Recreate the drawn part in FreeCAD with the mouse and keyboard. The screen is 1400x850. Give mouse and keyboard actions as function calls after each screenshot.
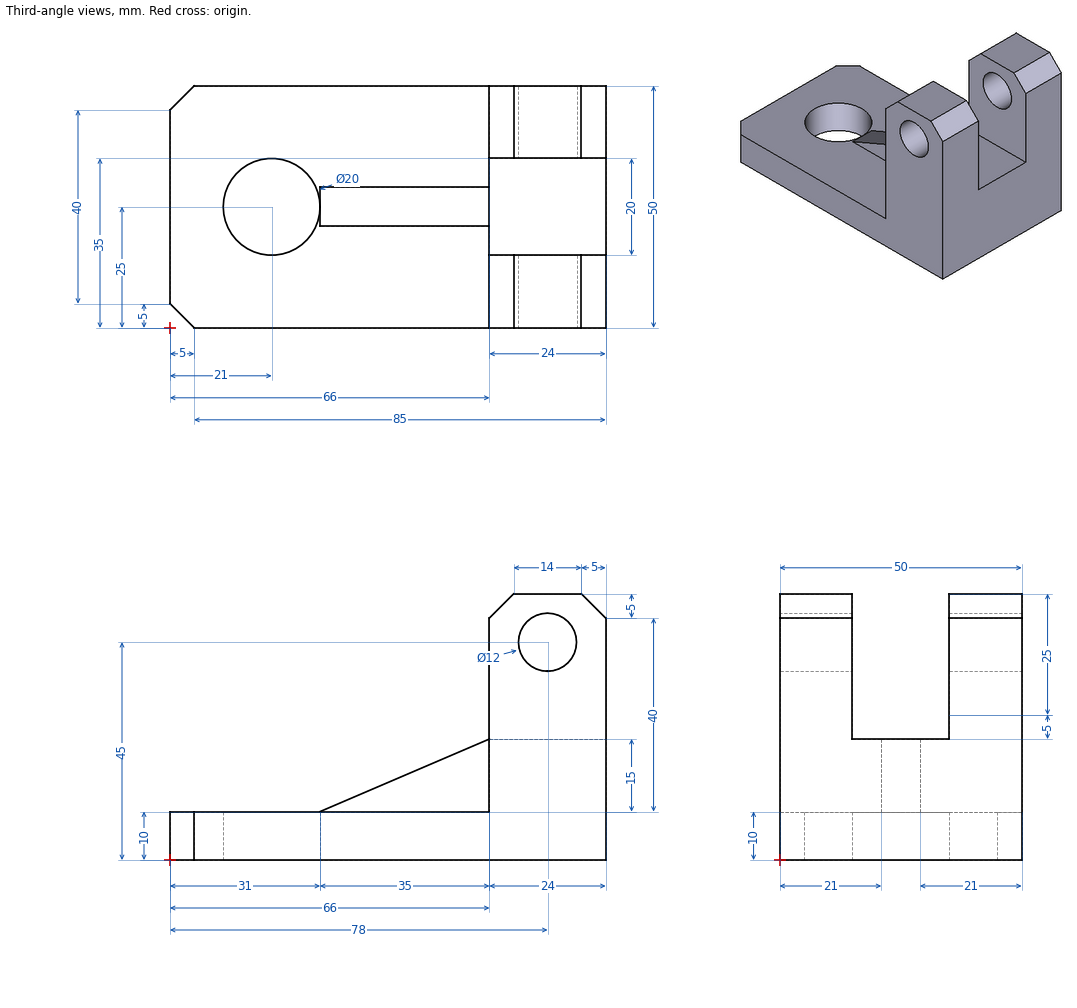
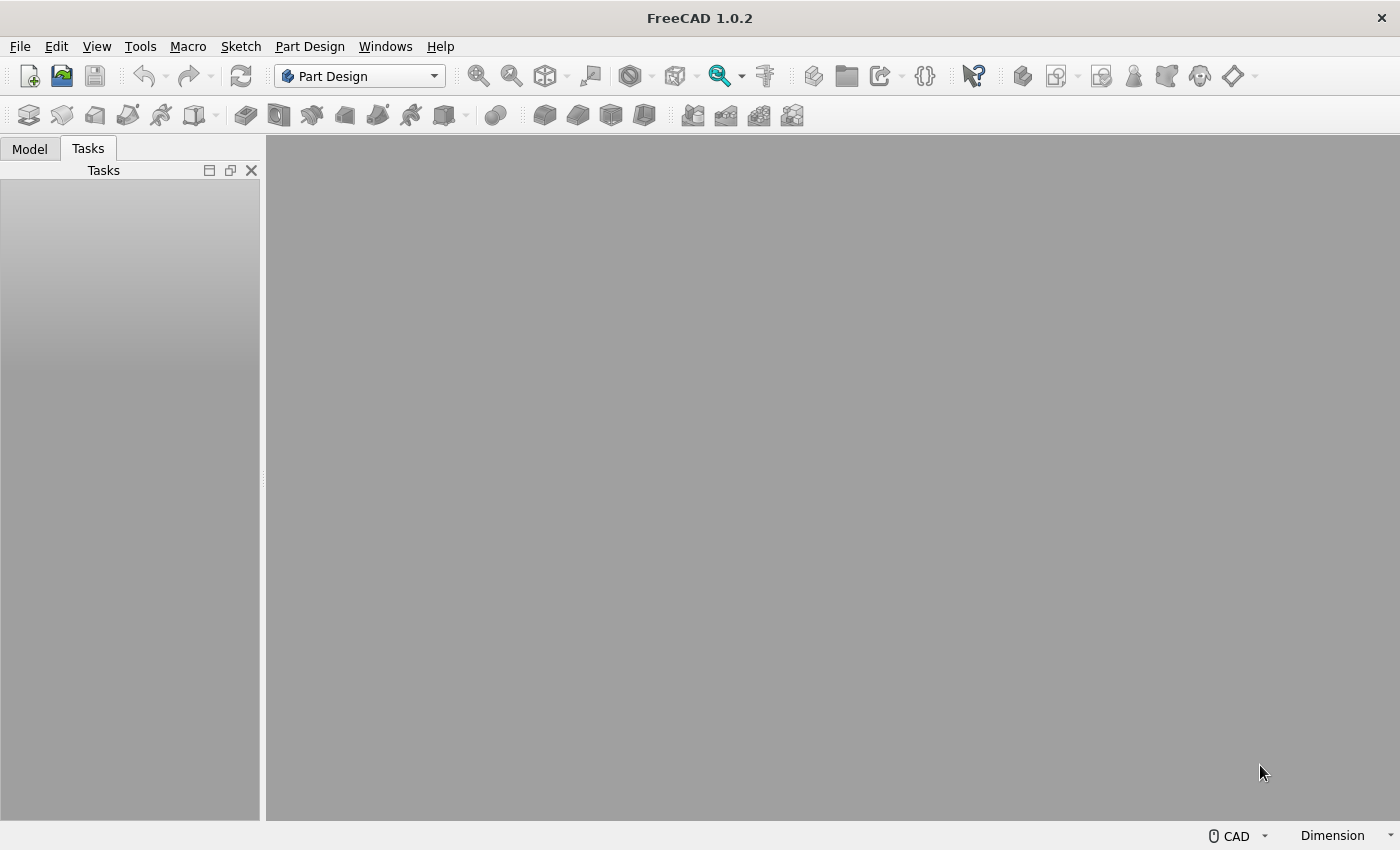
click(29, 76)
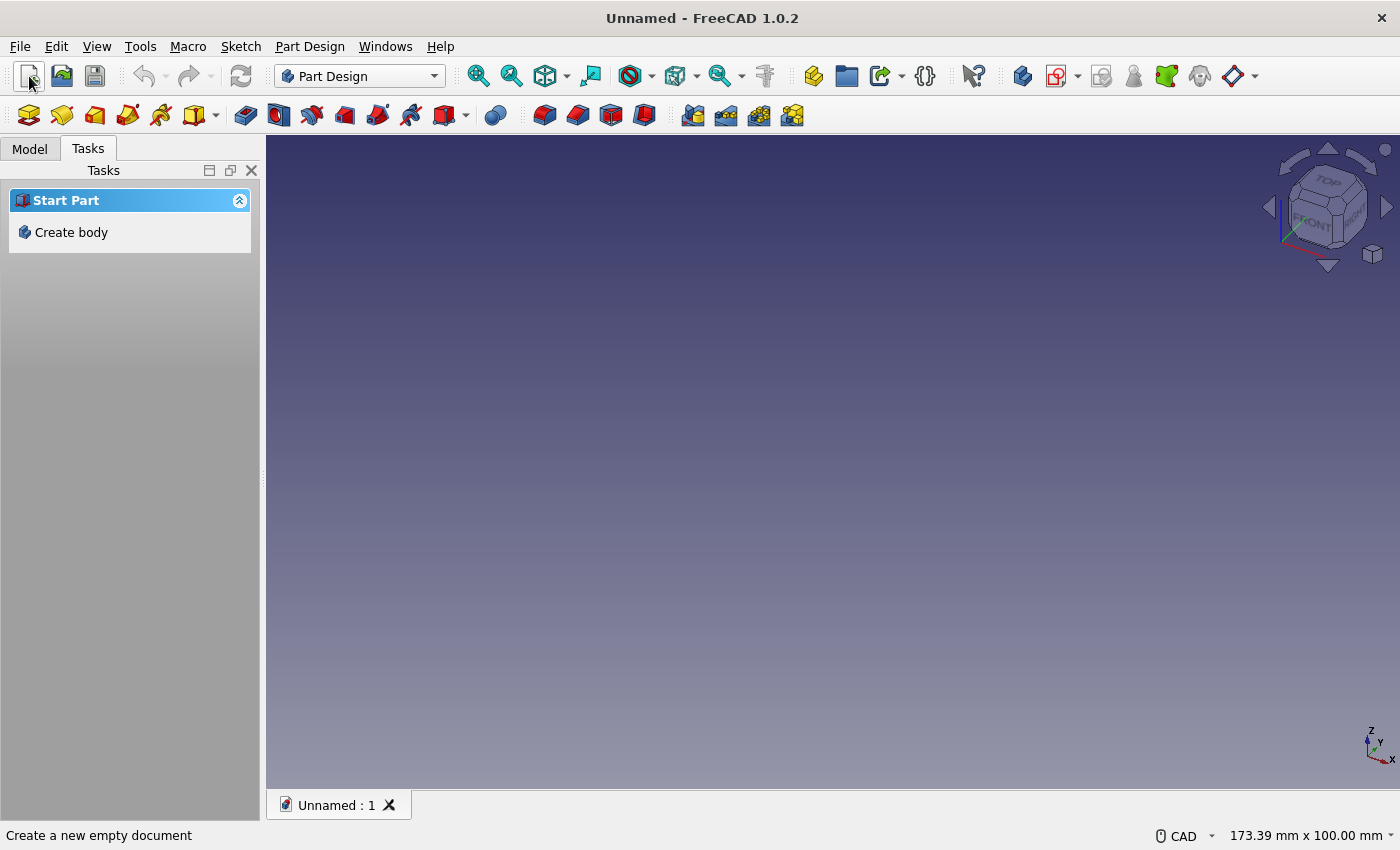
click(1056, 76)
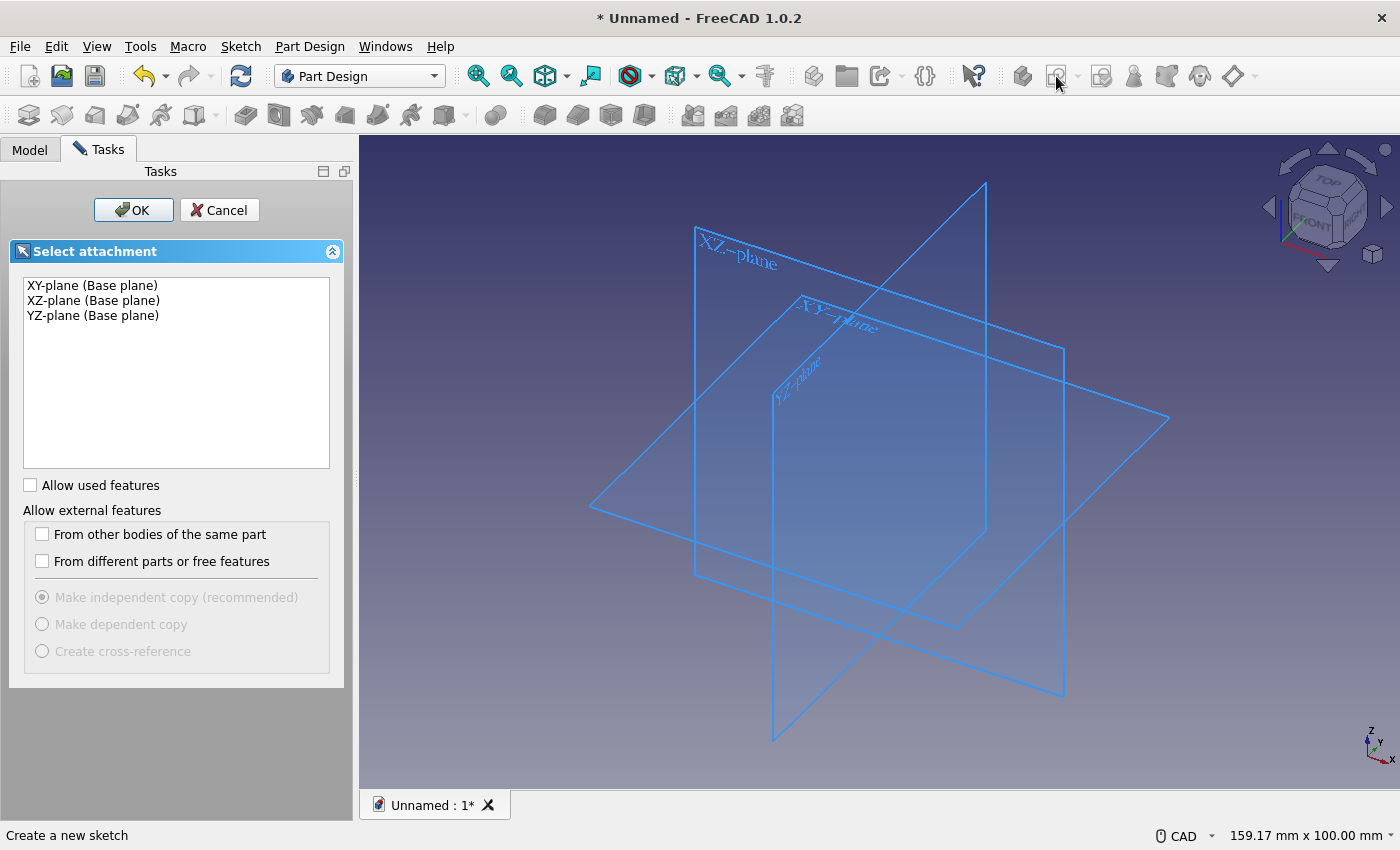
click(84, 286)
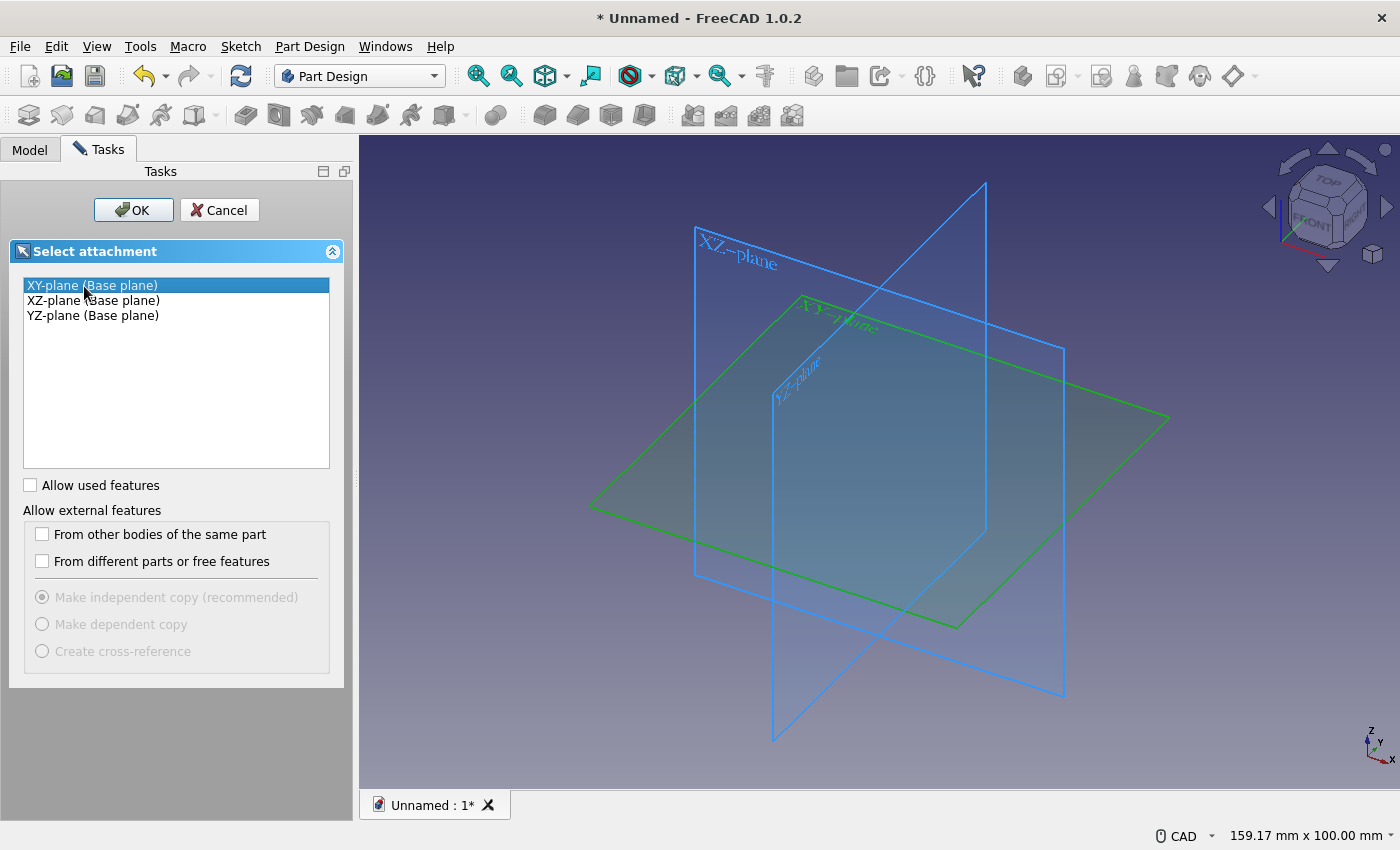
click(134, 210)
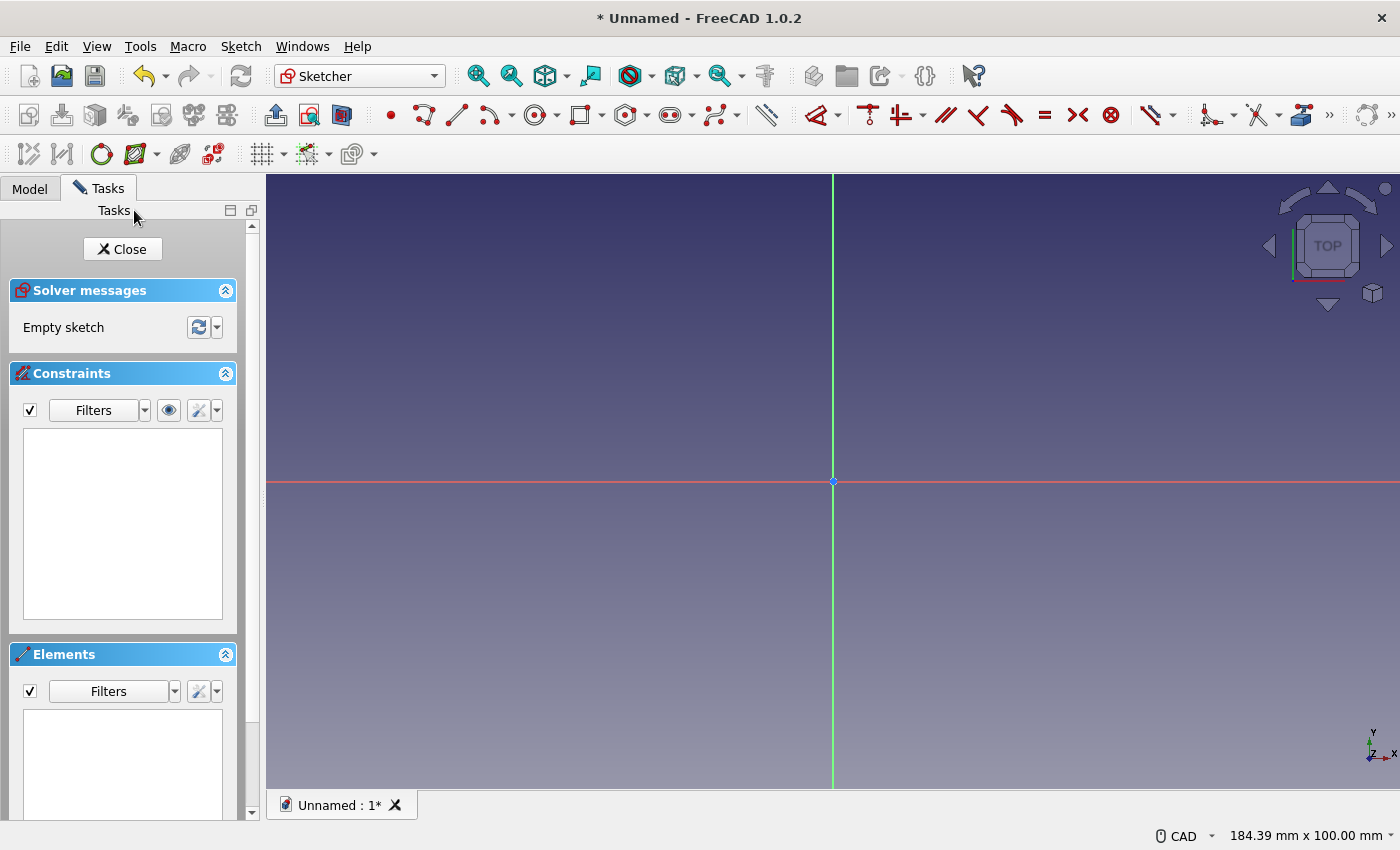
scroll(294, 761, down, 1)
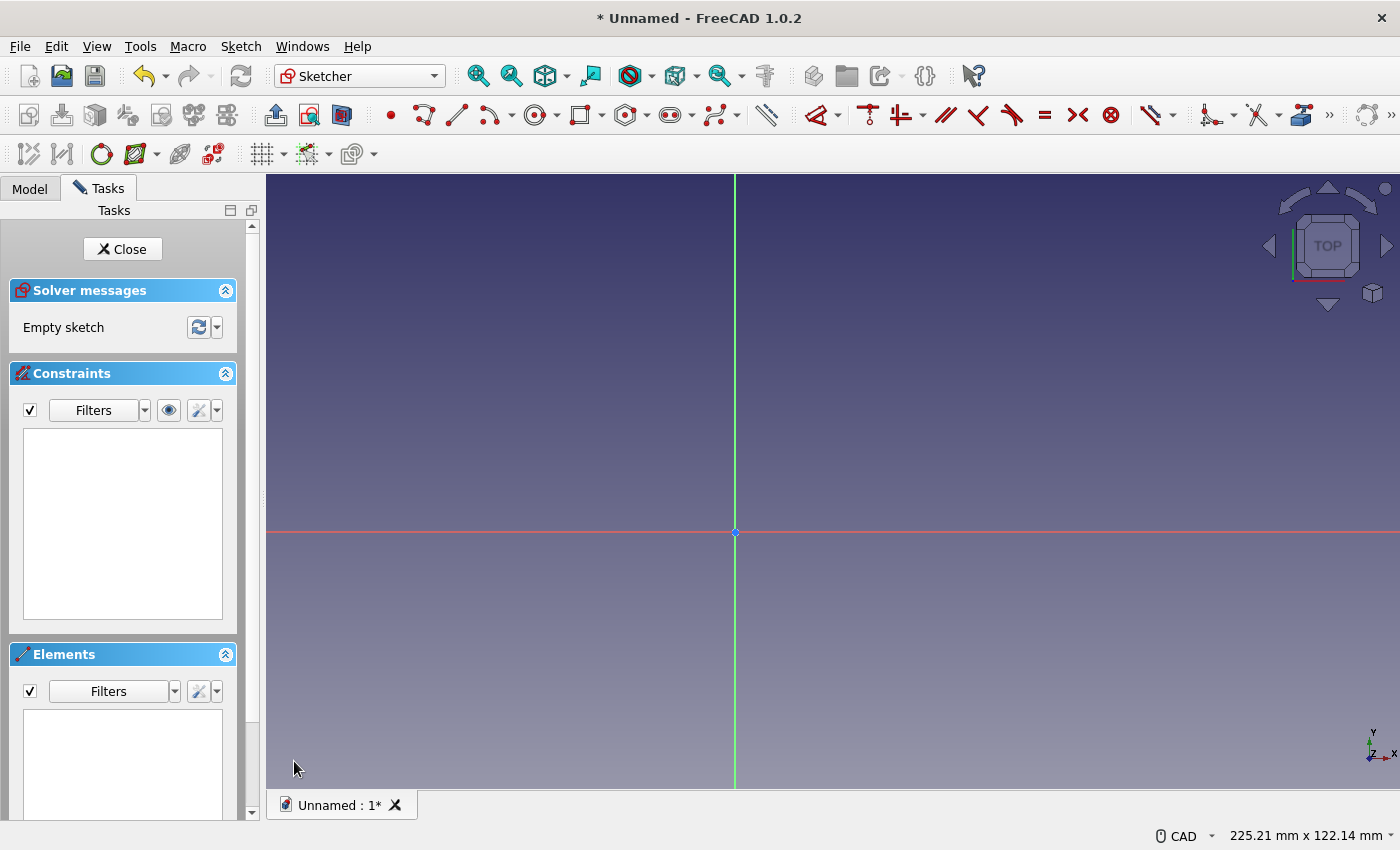
scroll(1235, 254, up, 2)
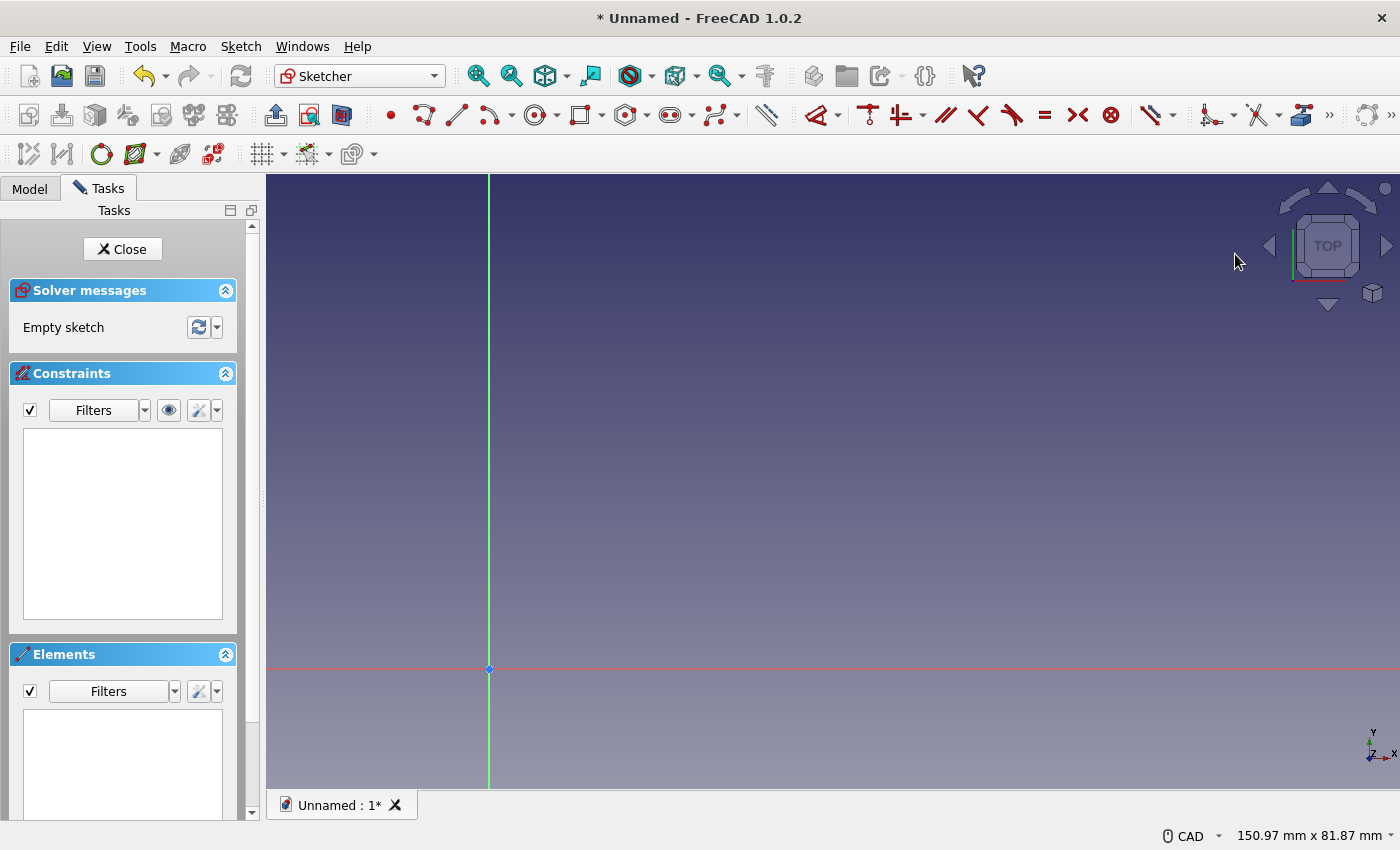
click(424, 116)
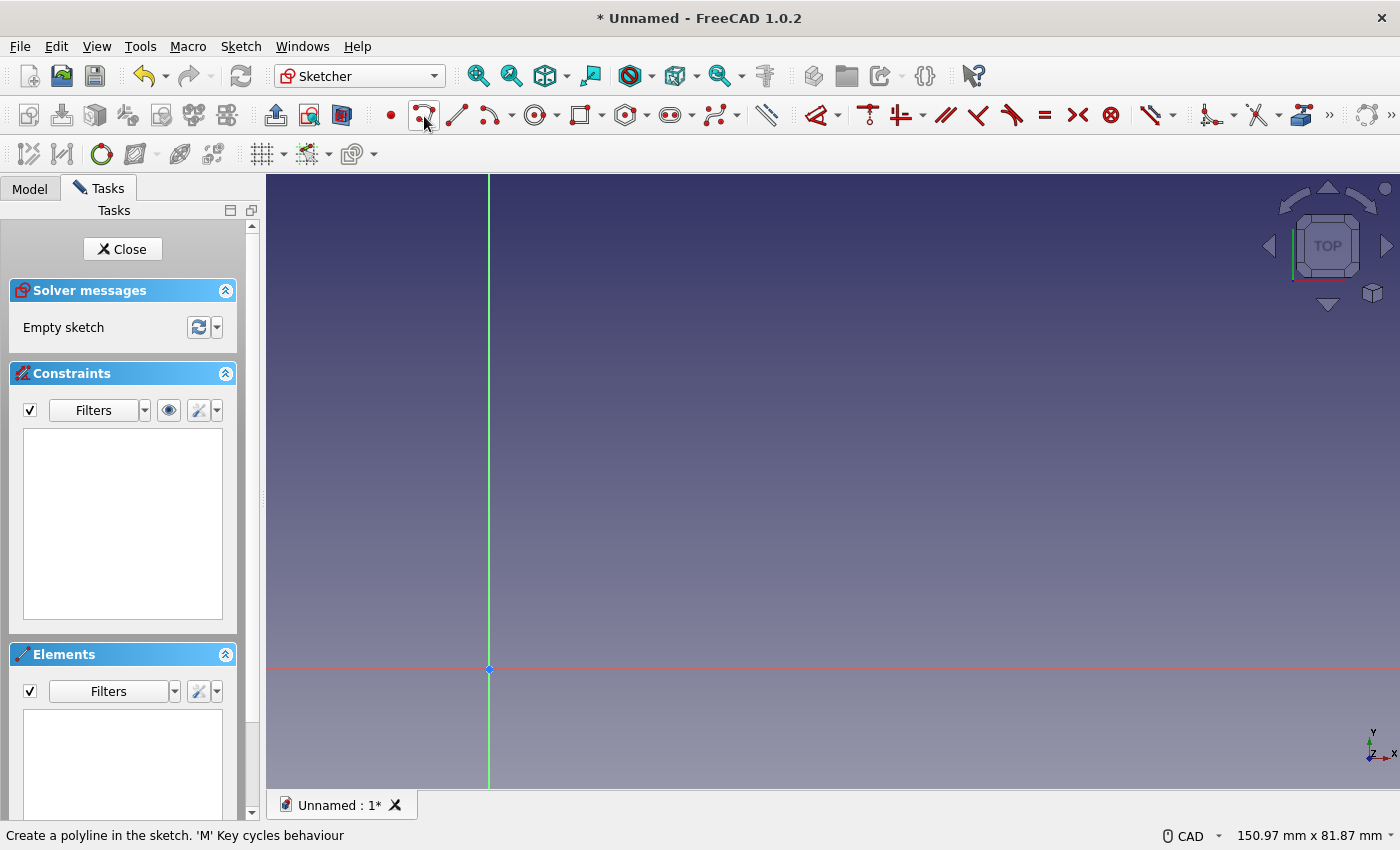
click(527, 669)
click(1165, 660)
click(1165, 294)
click(527, 294)
click(489, 331)
click(498, 632)
click(527, 669)
key(Escape)
key(Escape)